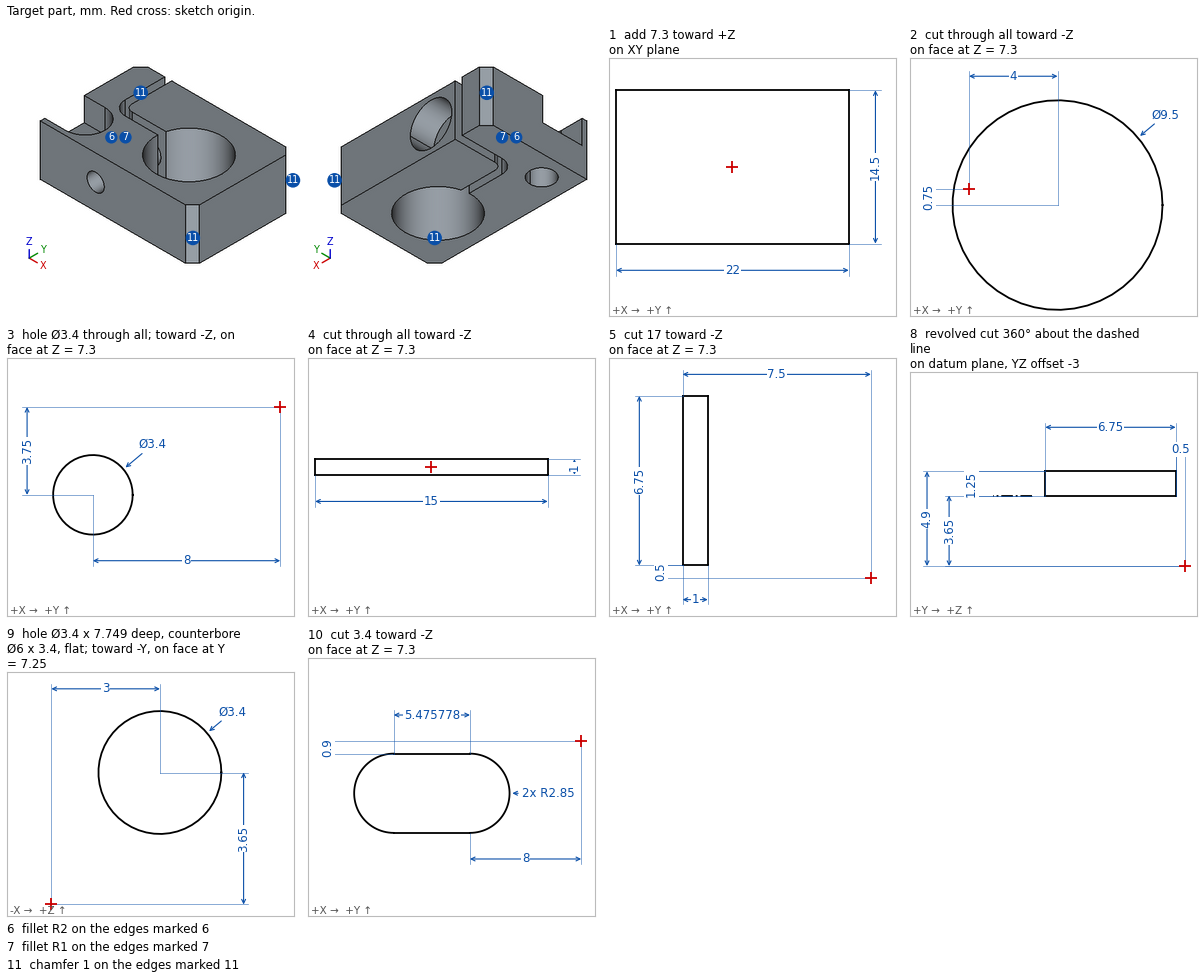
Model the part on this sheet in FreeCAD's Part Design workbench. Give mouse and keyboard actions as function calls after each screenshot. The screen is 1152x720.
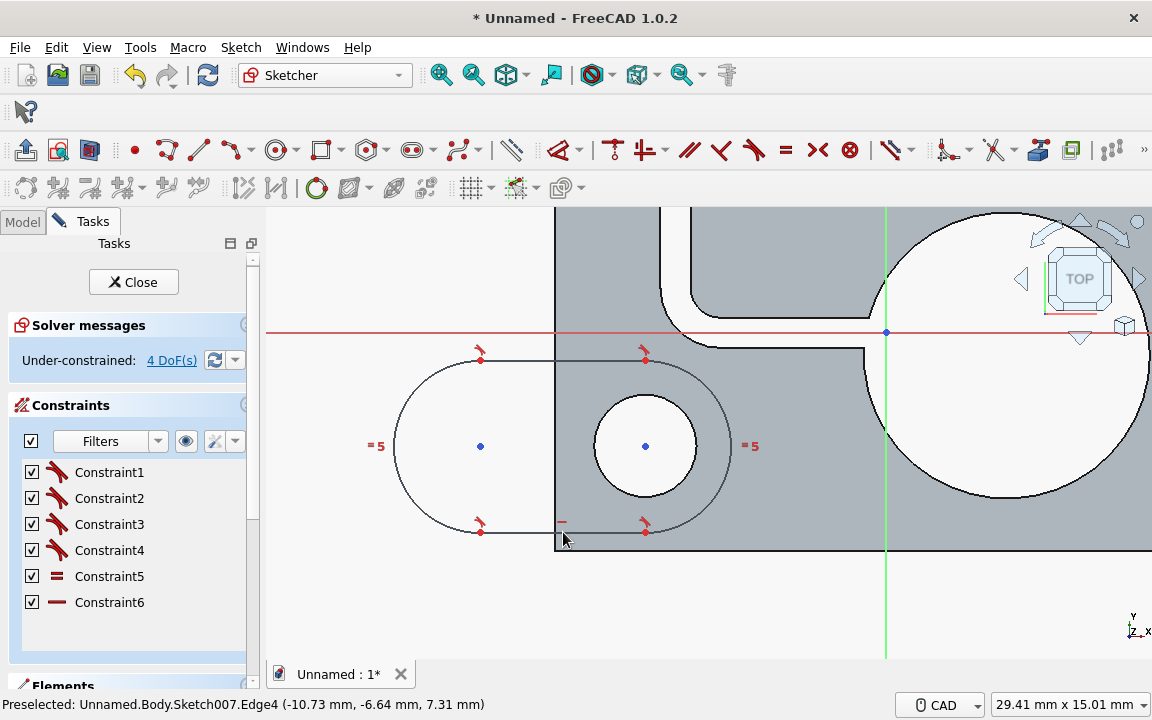
key(d)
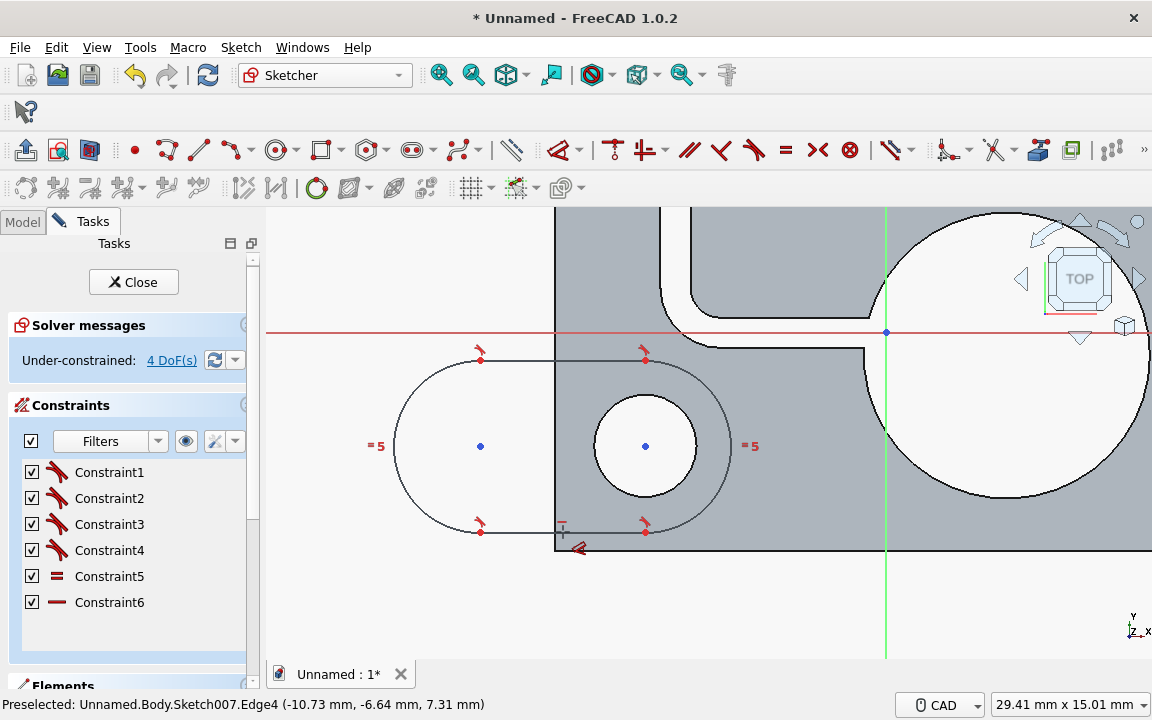
click(410, 396)
click(384, 377)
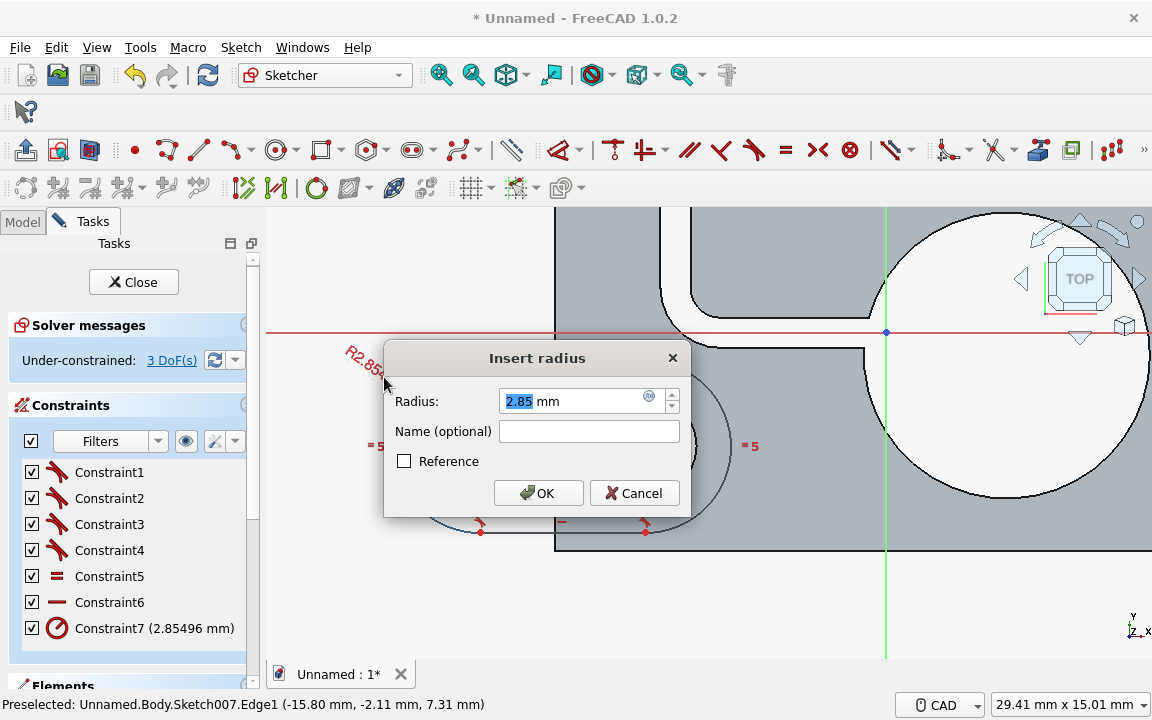
text(2.85)
key(Return)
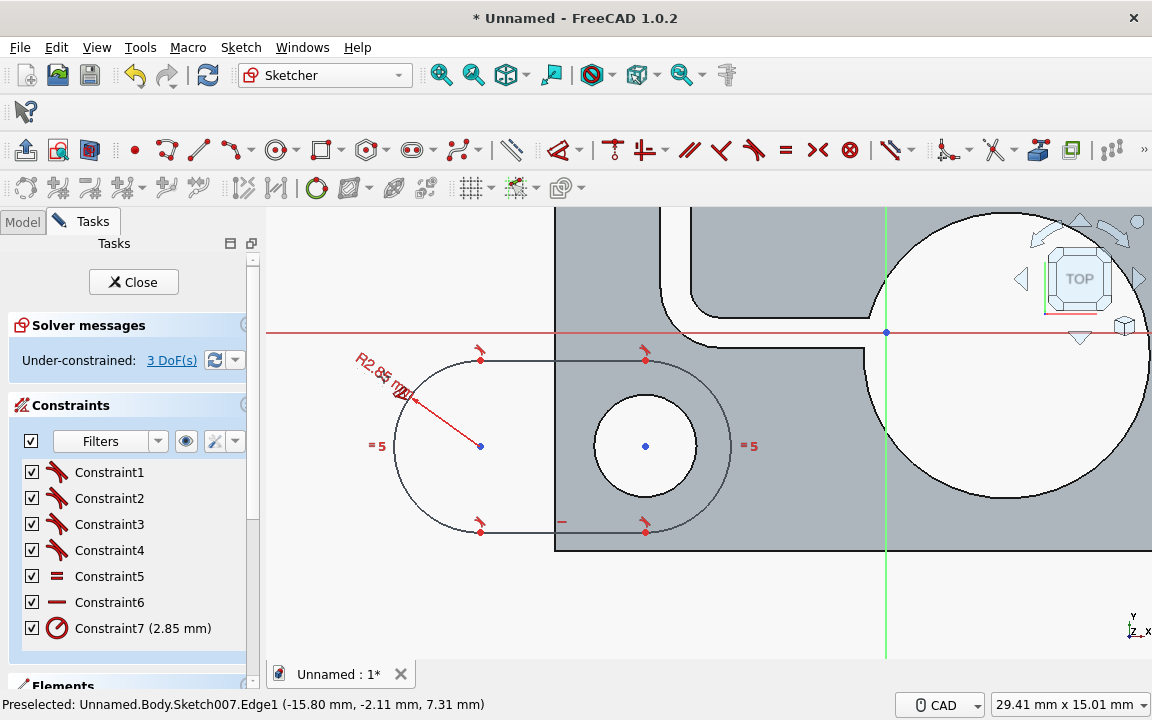
click(645, 533)
click(766, 567)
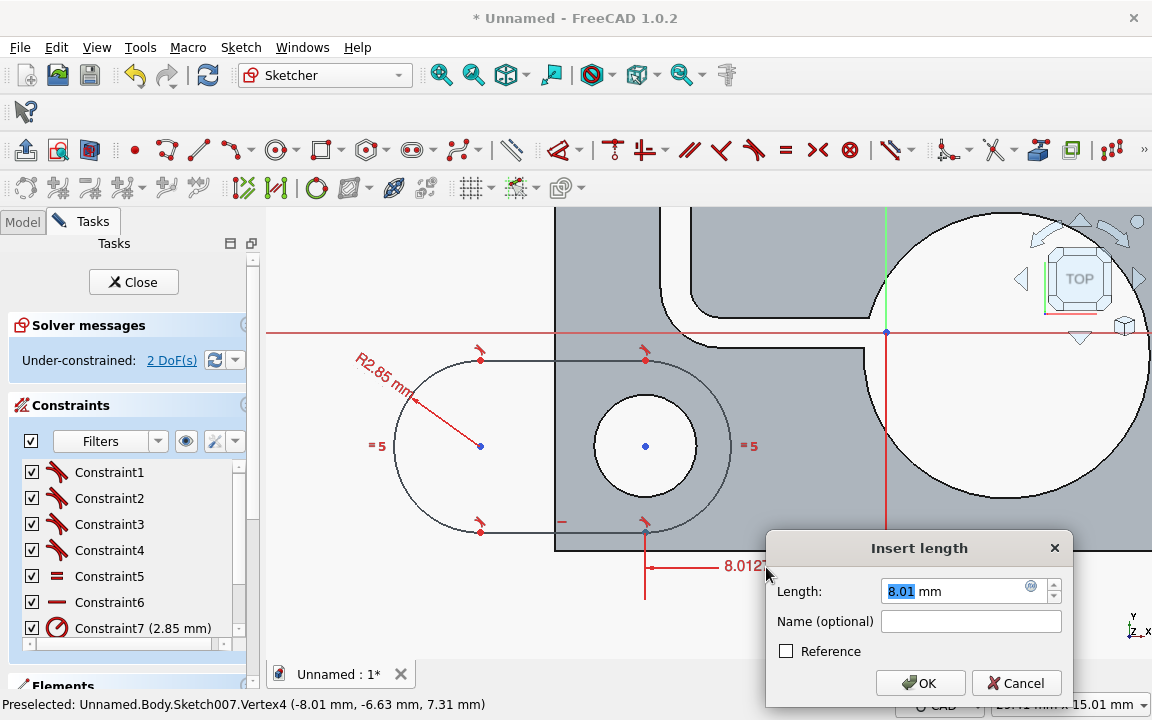
text(8)
key(Return)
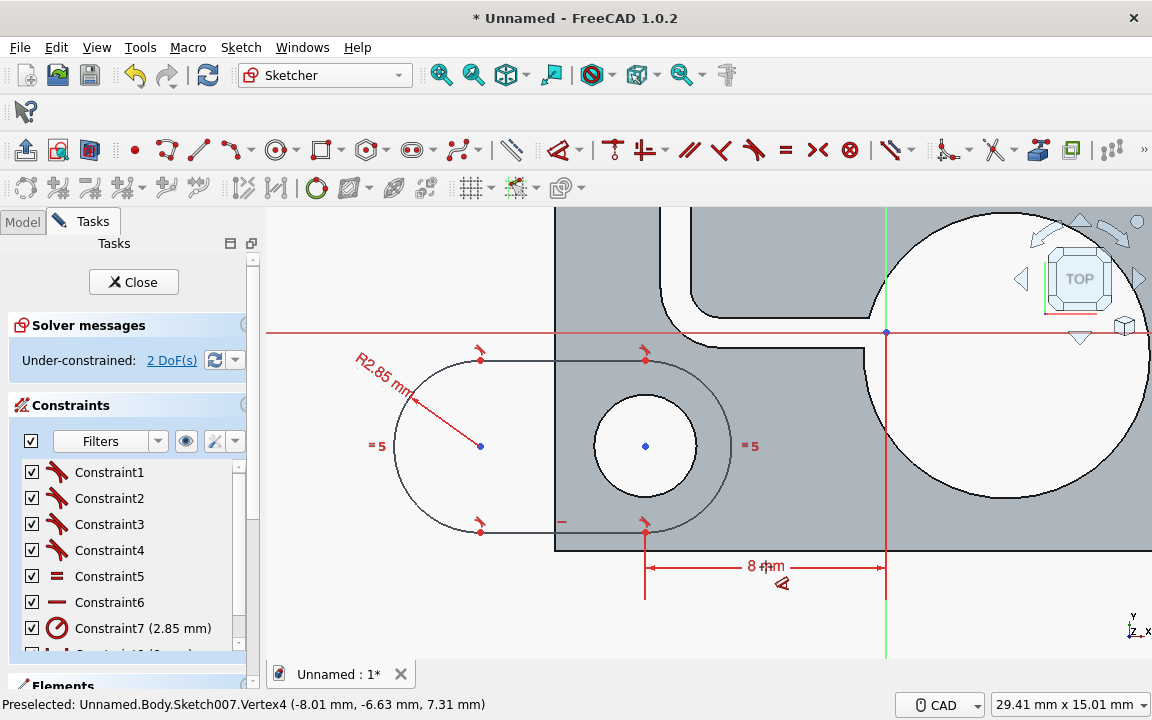
scroll(480, 361, up, 2)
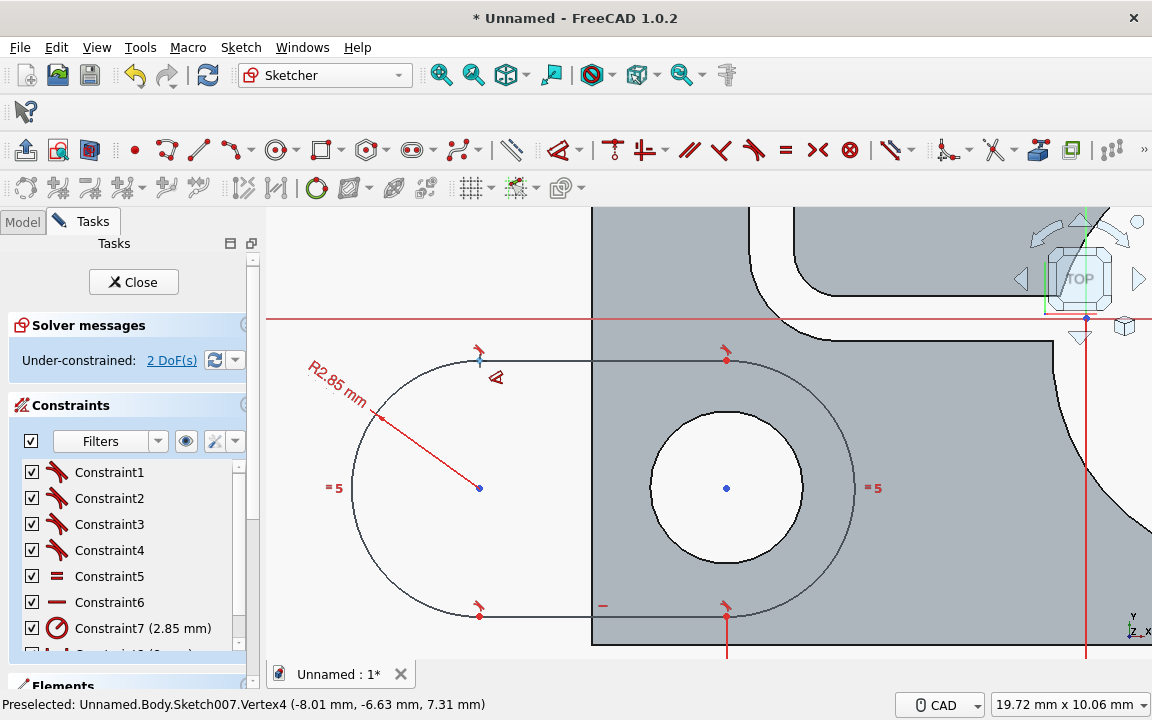
click(480, 361)
click(446, 340)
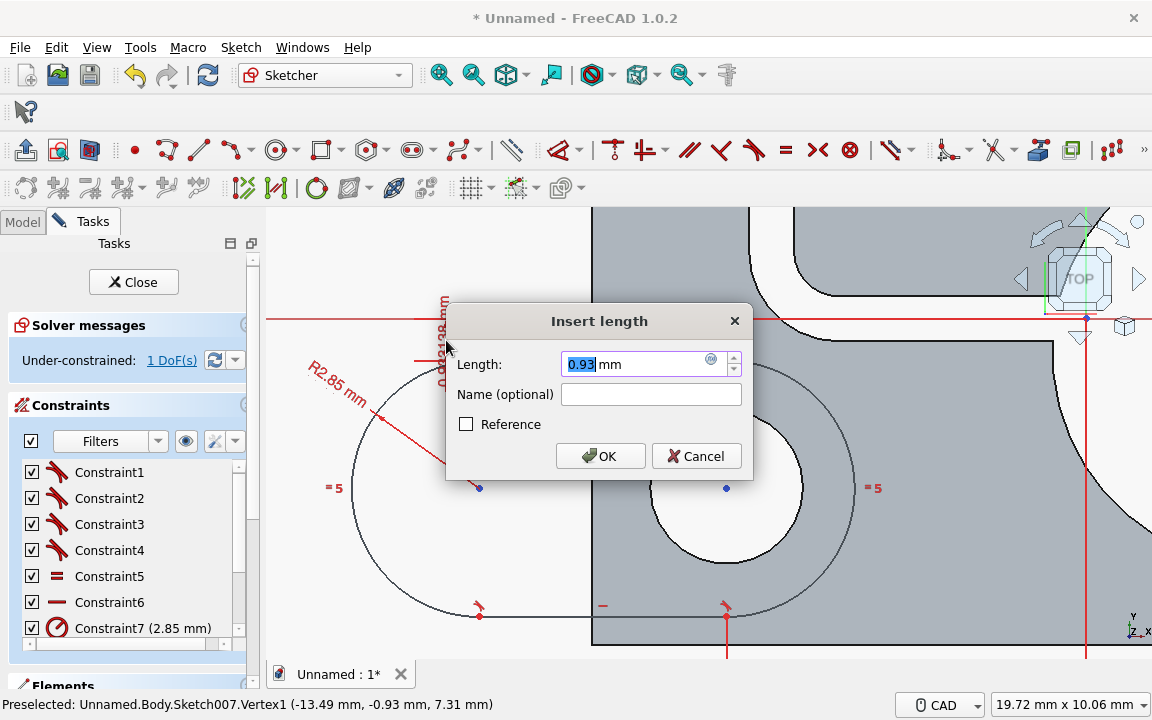
text(0.9)
key(Return)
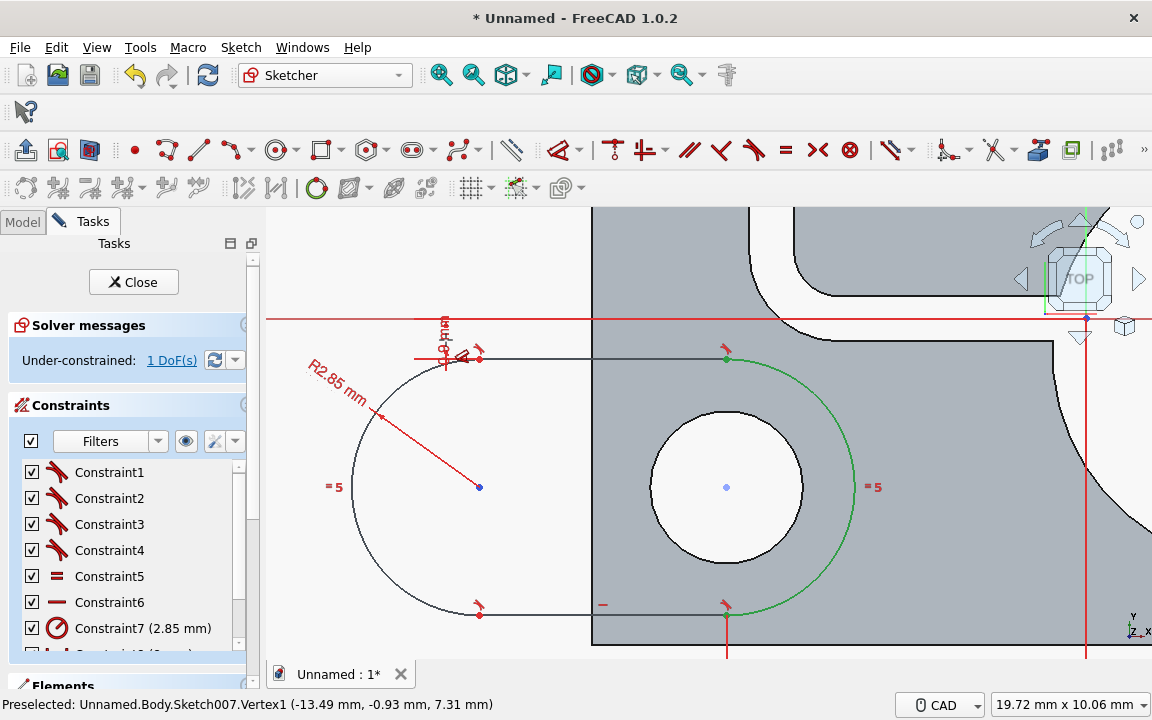
click(554, 359)
click(603, 393)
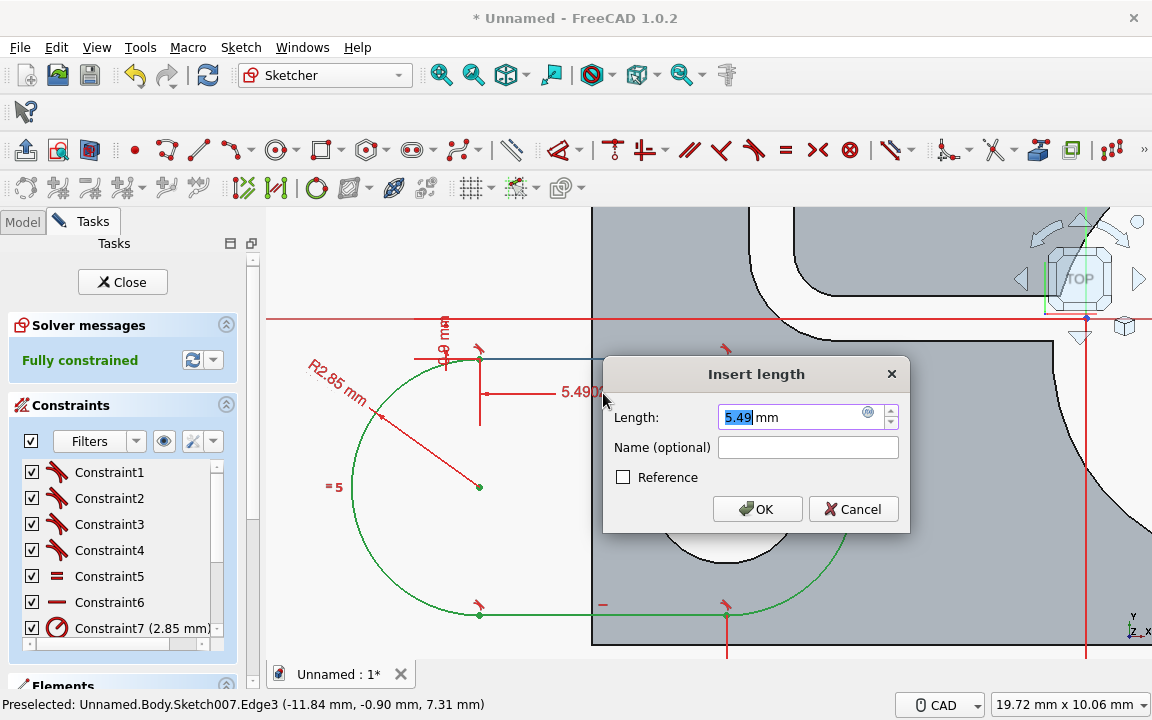
text(5.475778)
key(Return)
key(Escape)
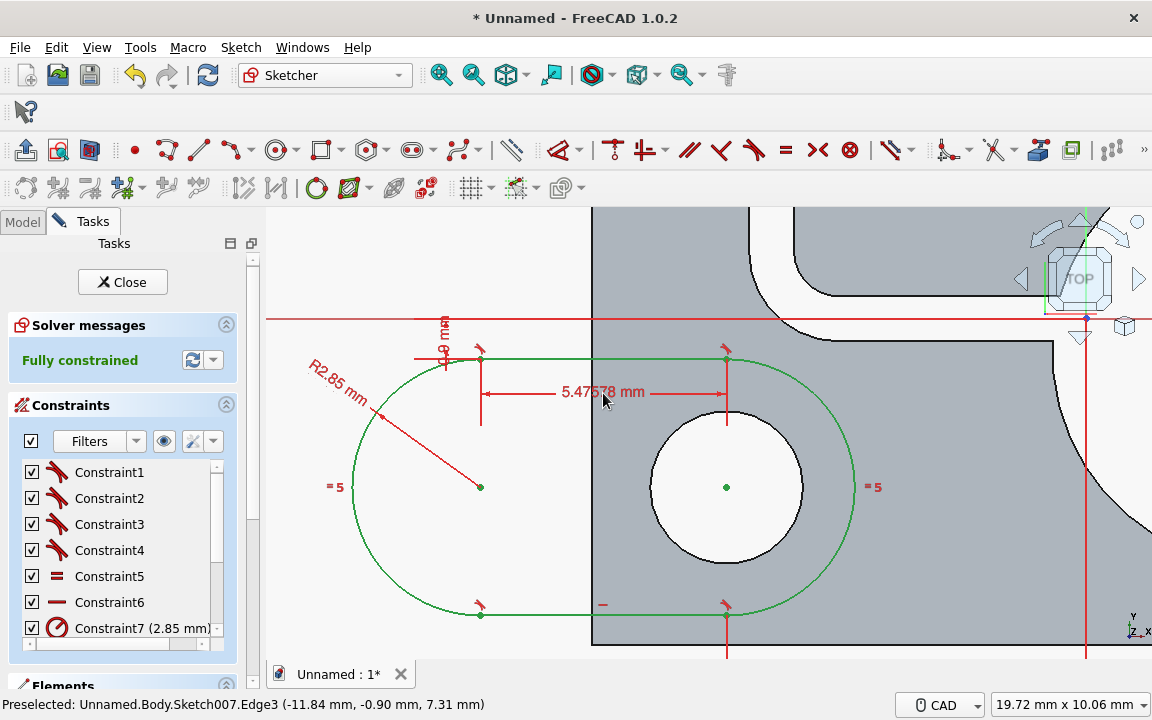
click(123, 282)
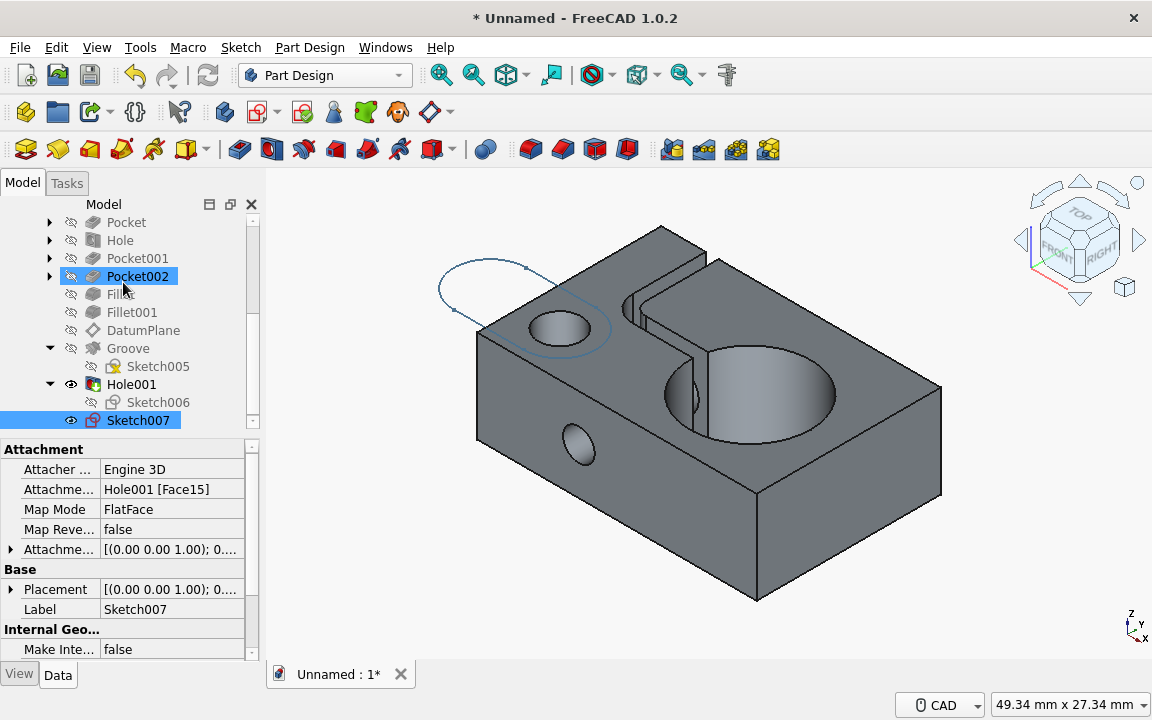
click(240, 150)